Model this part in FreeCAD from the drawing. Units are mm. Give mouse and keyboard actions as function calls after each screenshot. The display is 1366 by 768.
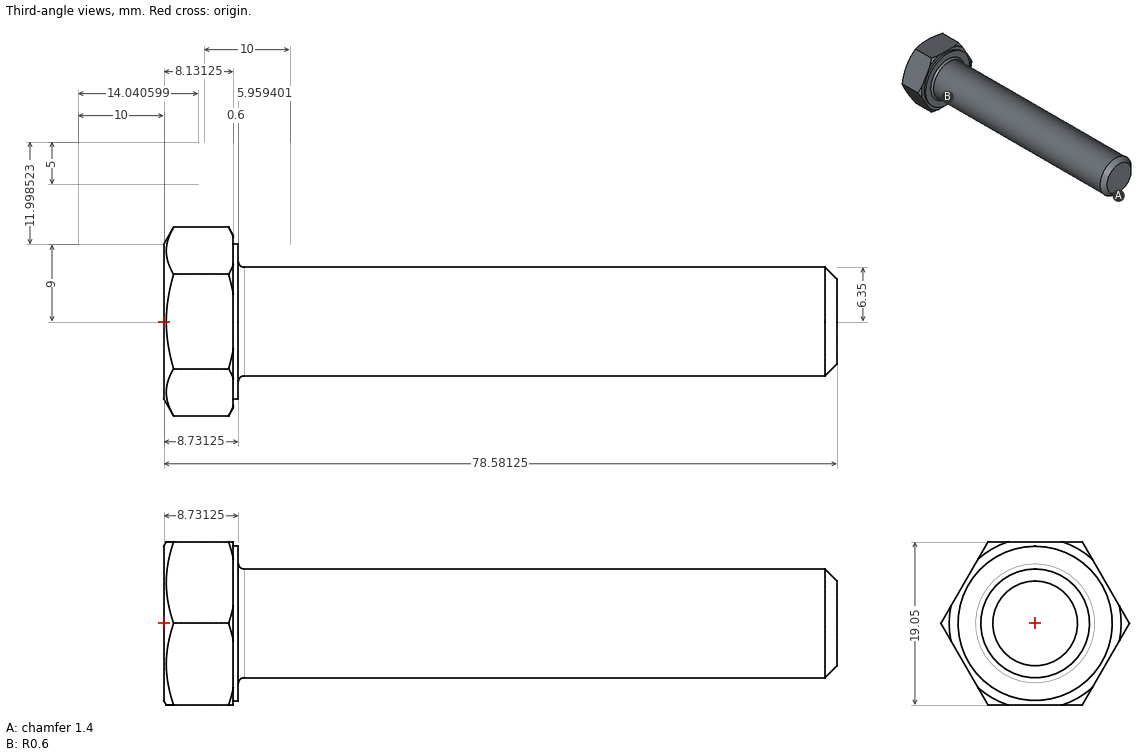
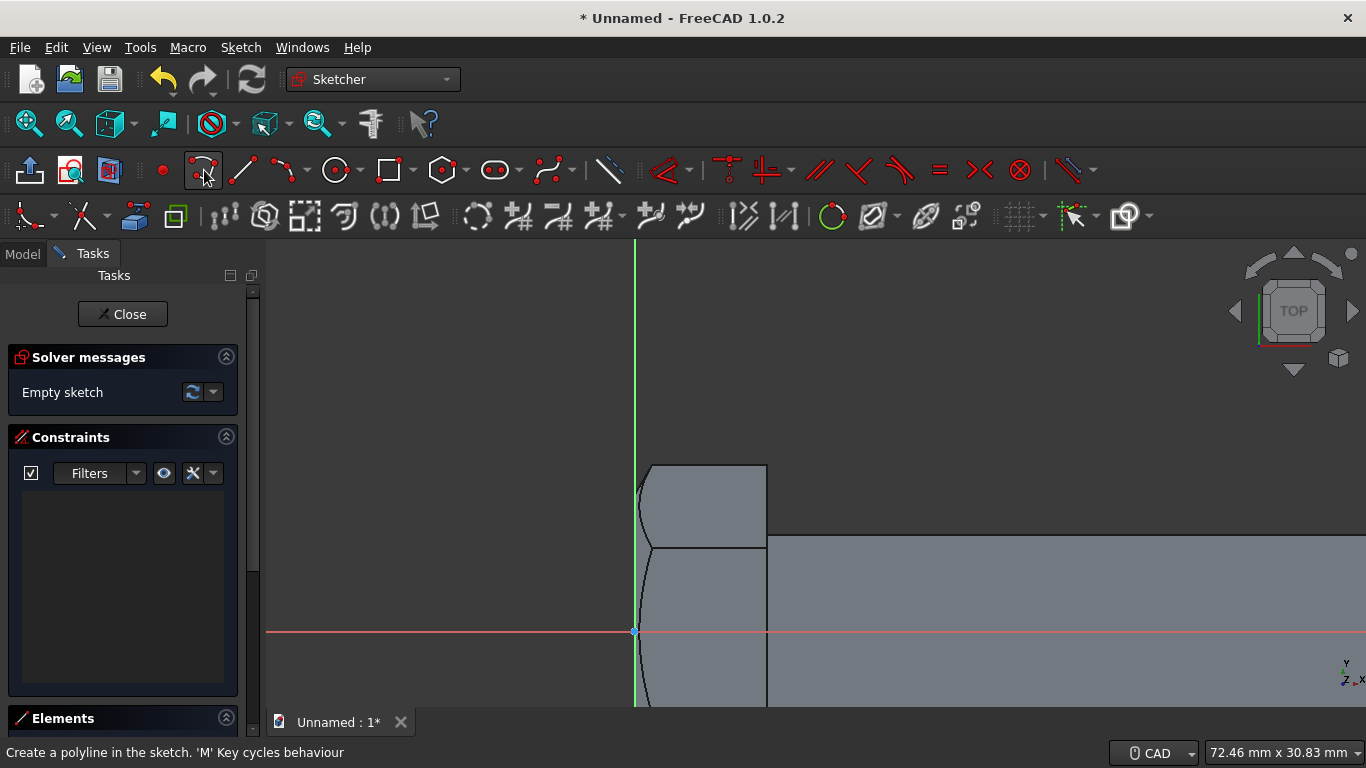
click(767, 495)
click(858, 495)
click(858, 313)
click(706, 313)
click(706, 389)
click(767, 496)
key(Escape)
key(Escape)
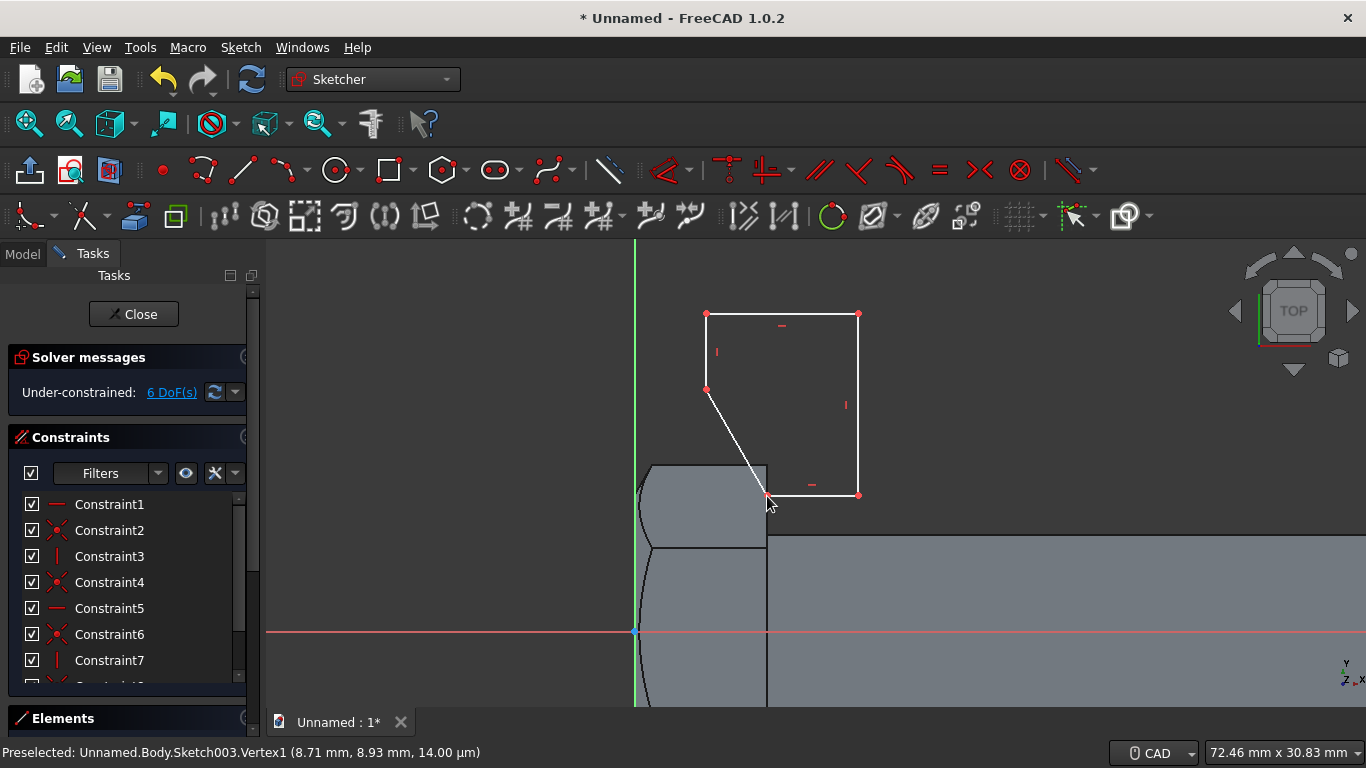
click(664, 170)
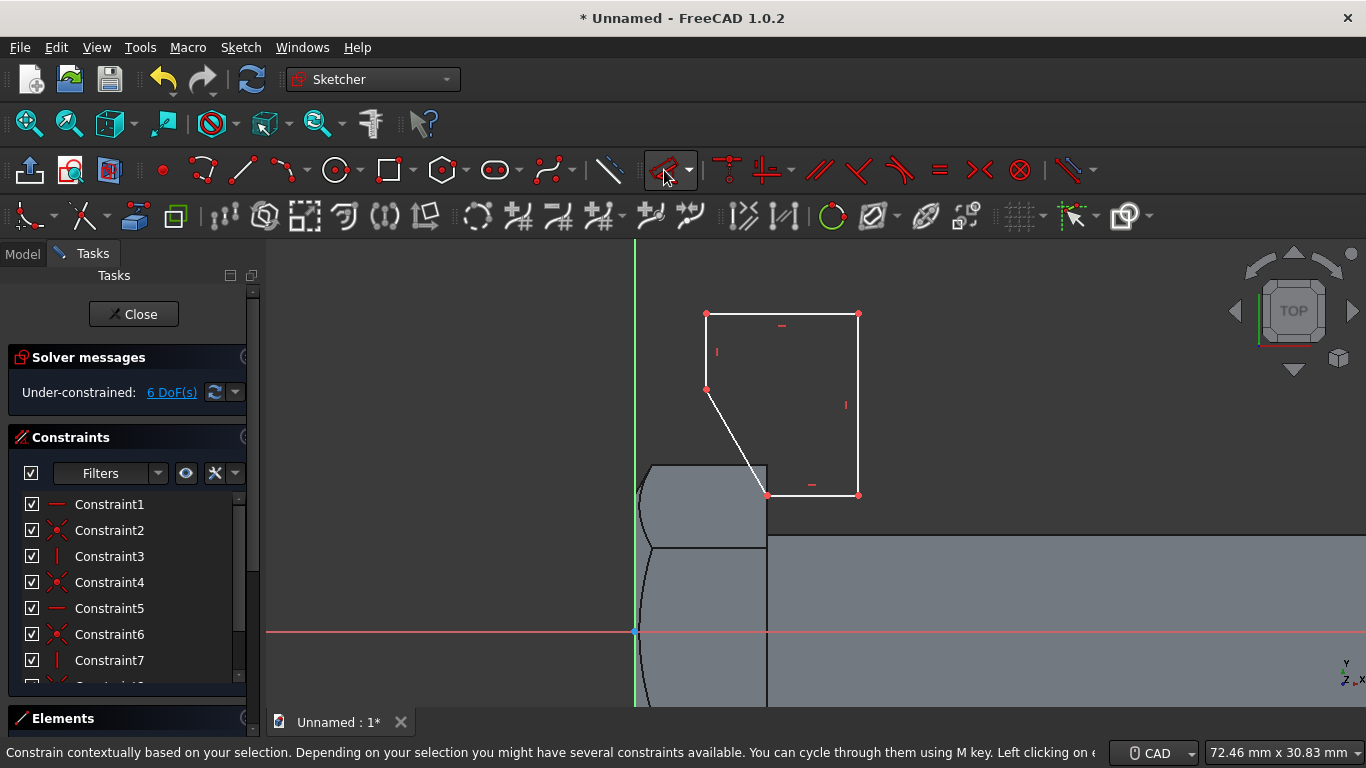
click(706, 337)
click(672, 352)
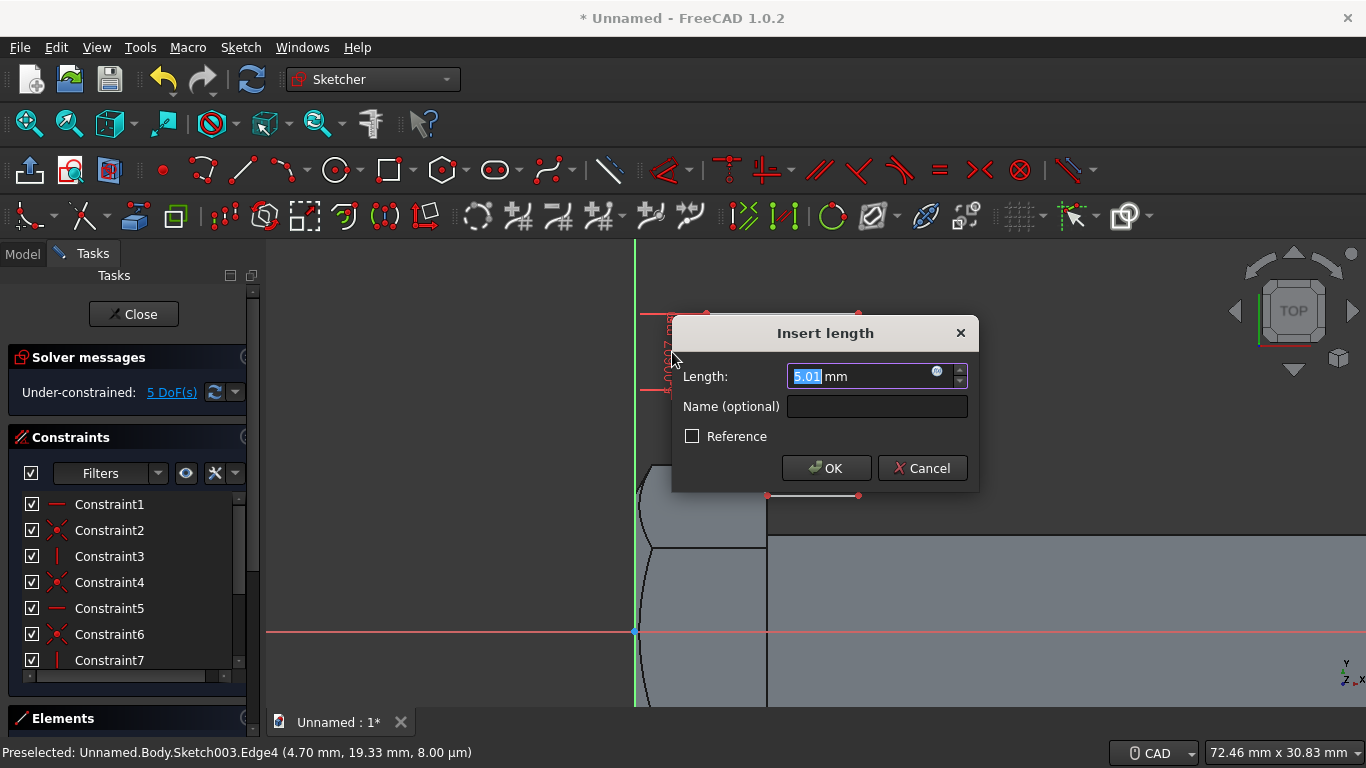
text(5)
key(Return)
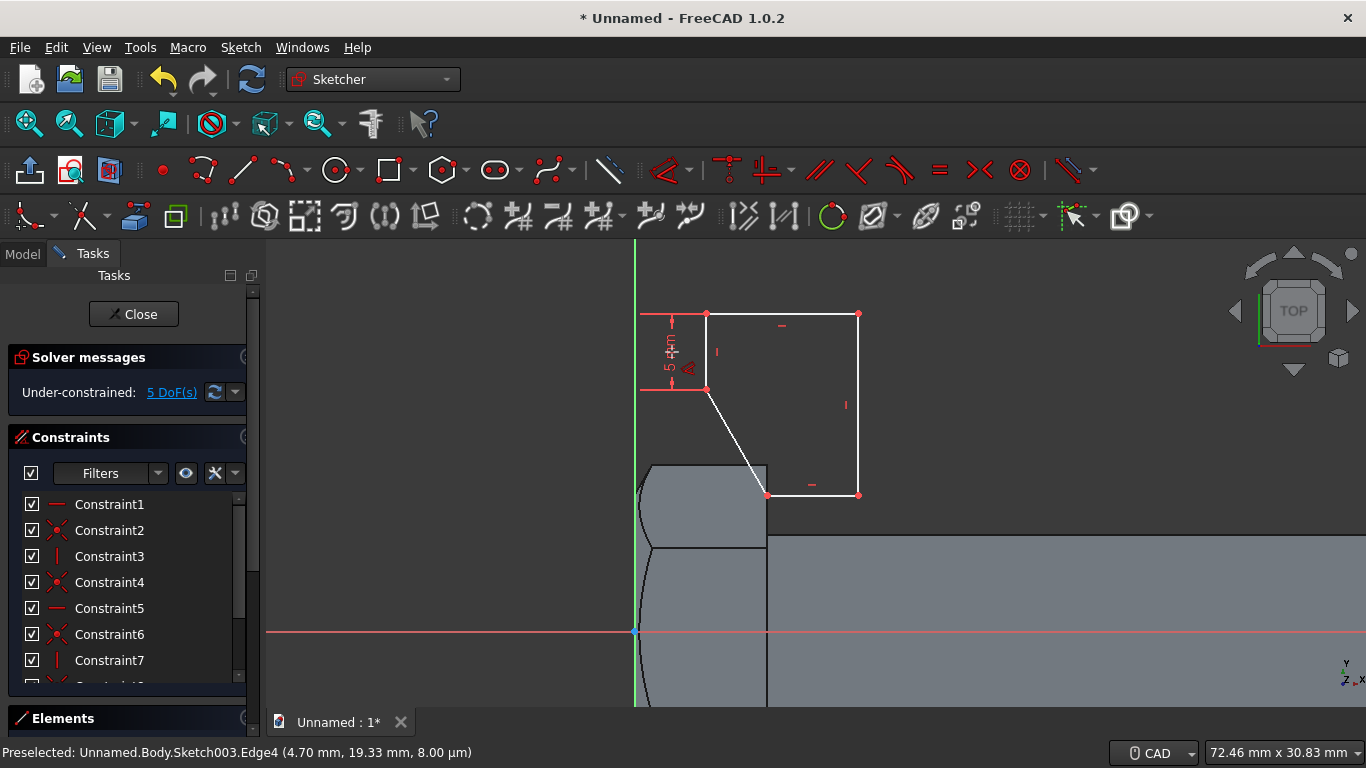
click(812, 314)
click(782, 280)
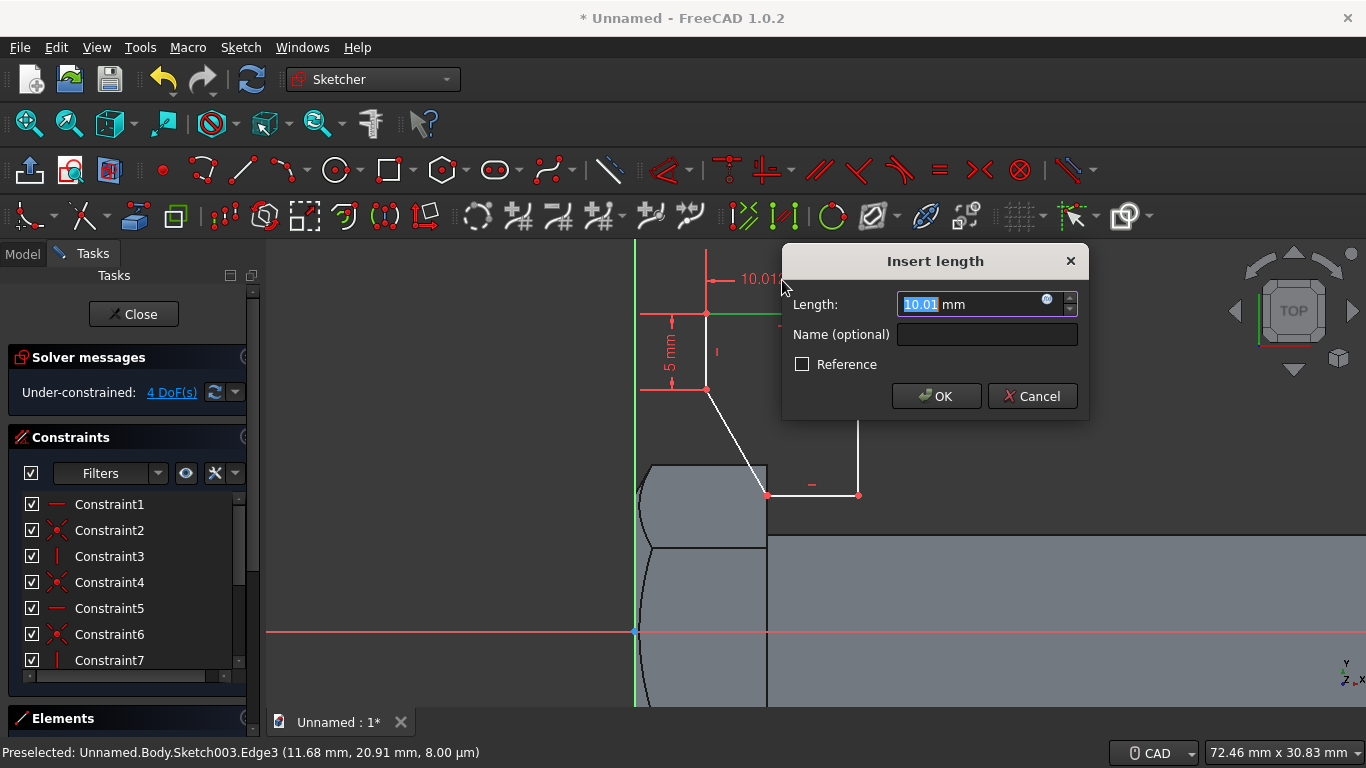
text(10)
key(Return)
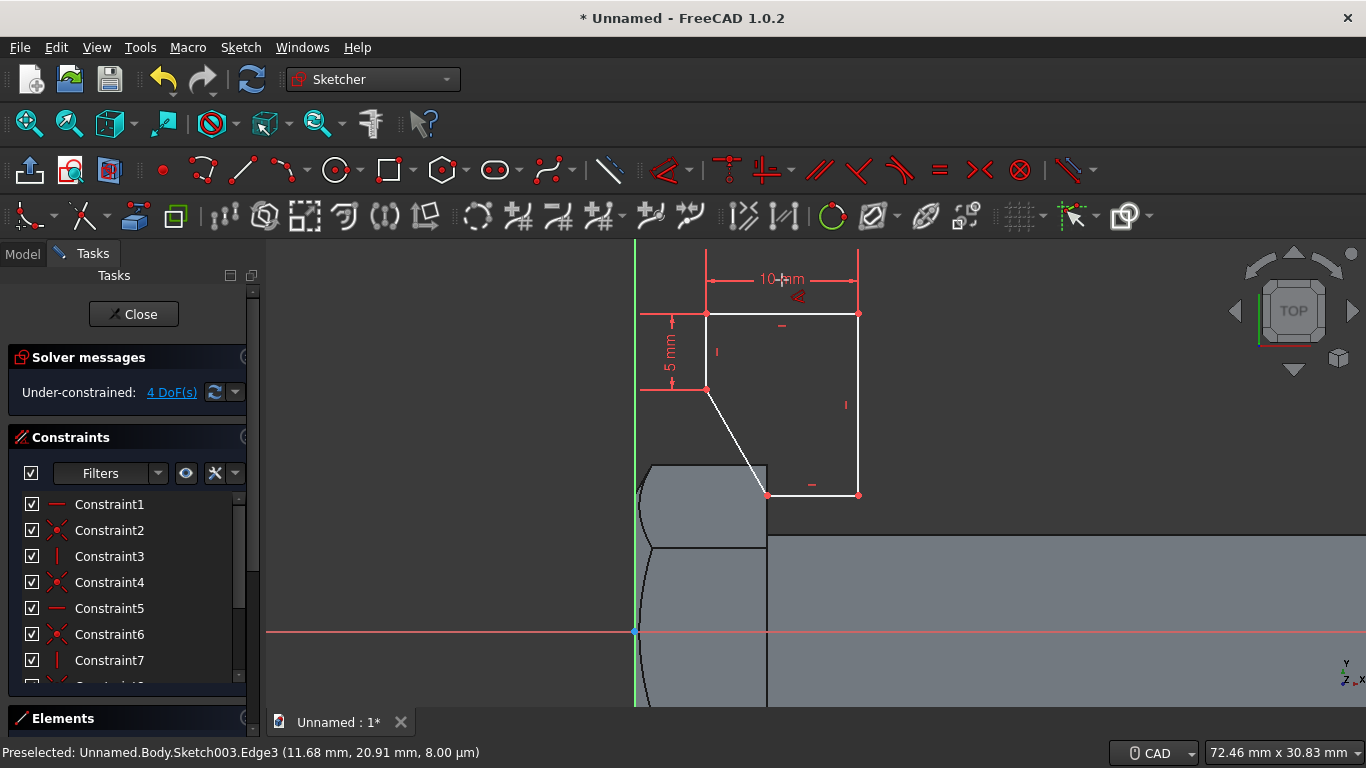
click(767, 496)
click(601, 564)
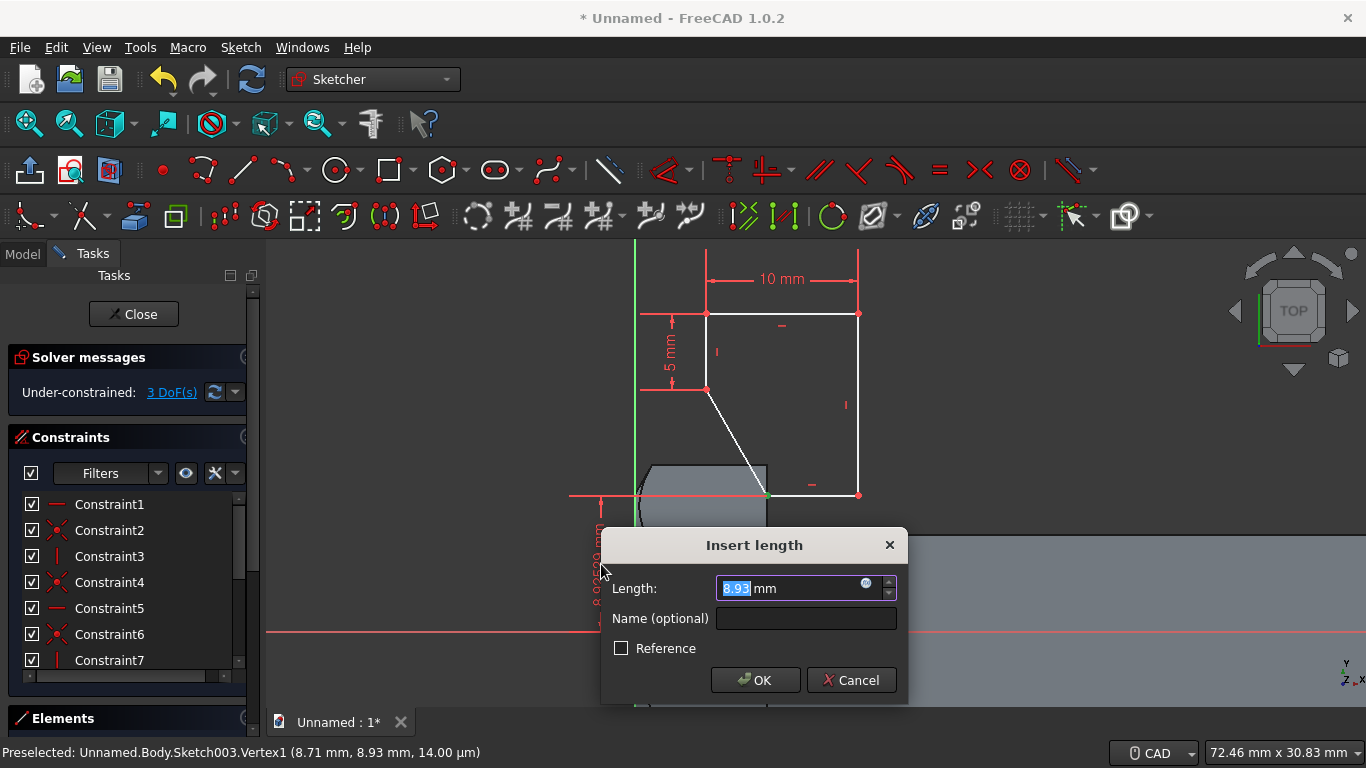
text(9)
key(Return)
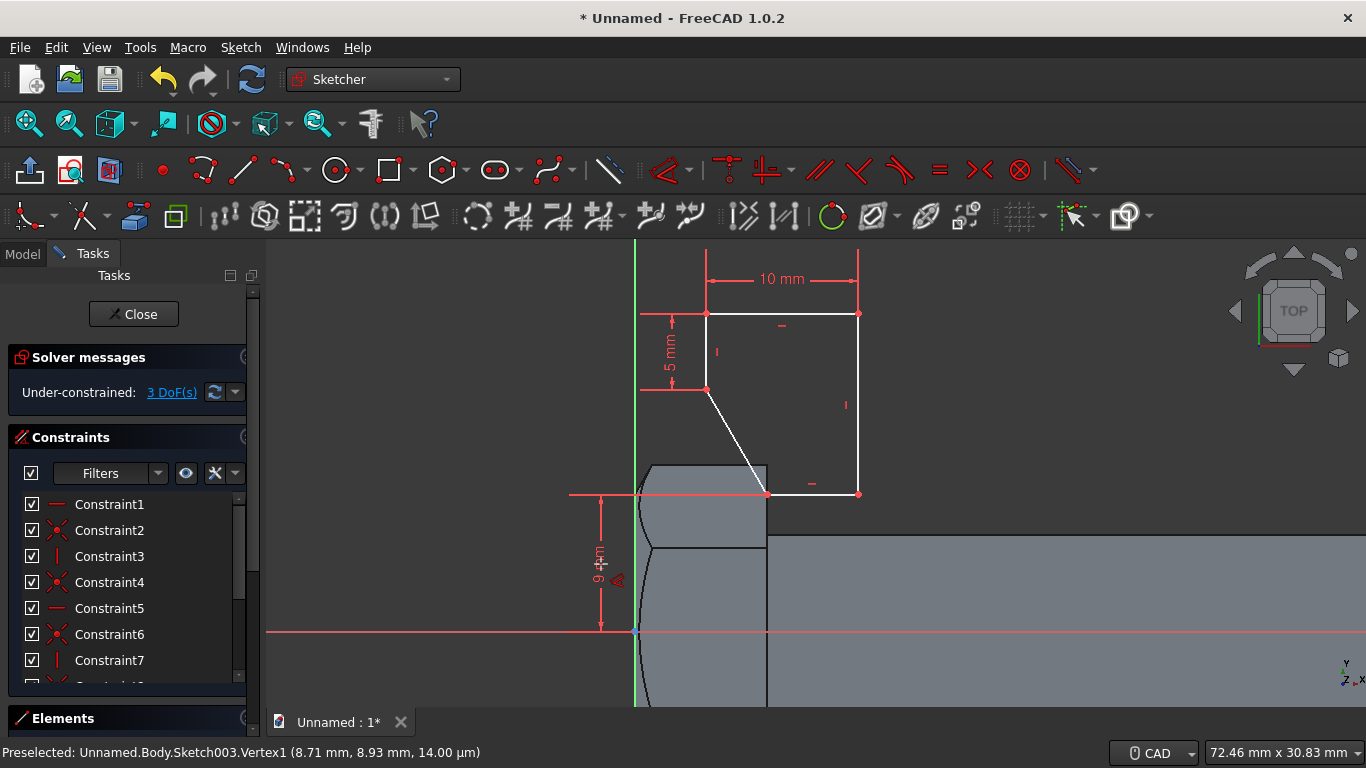
click(794, 495)
click(813, 529)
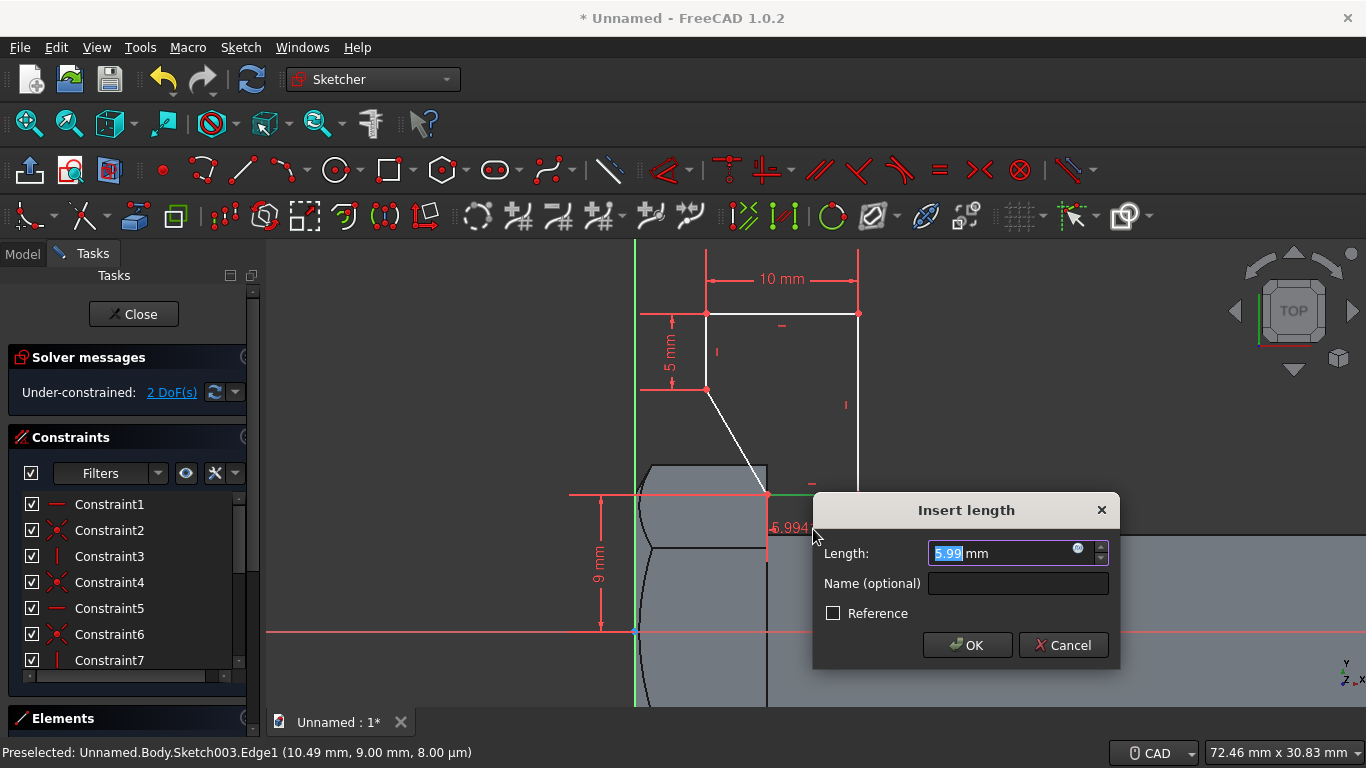
text(5.959401)
key(Return)